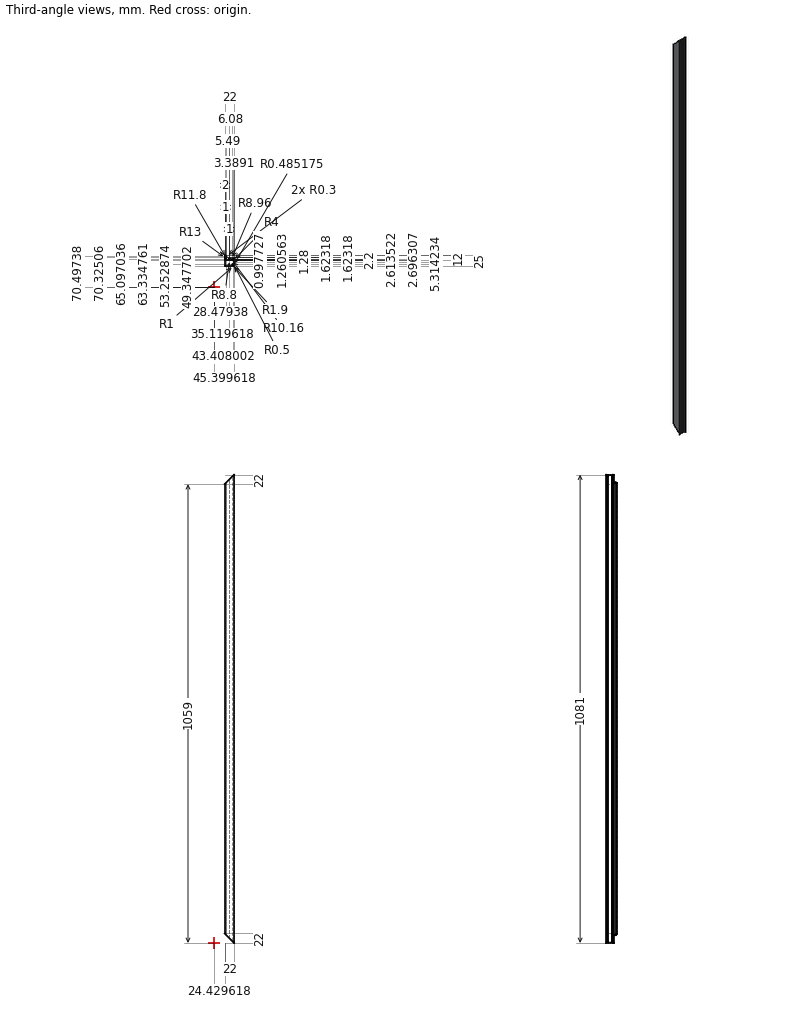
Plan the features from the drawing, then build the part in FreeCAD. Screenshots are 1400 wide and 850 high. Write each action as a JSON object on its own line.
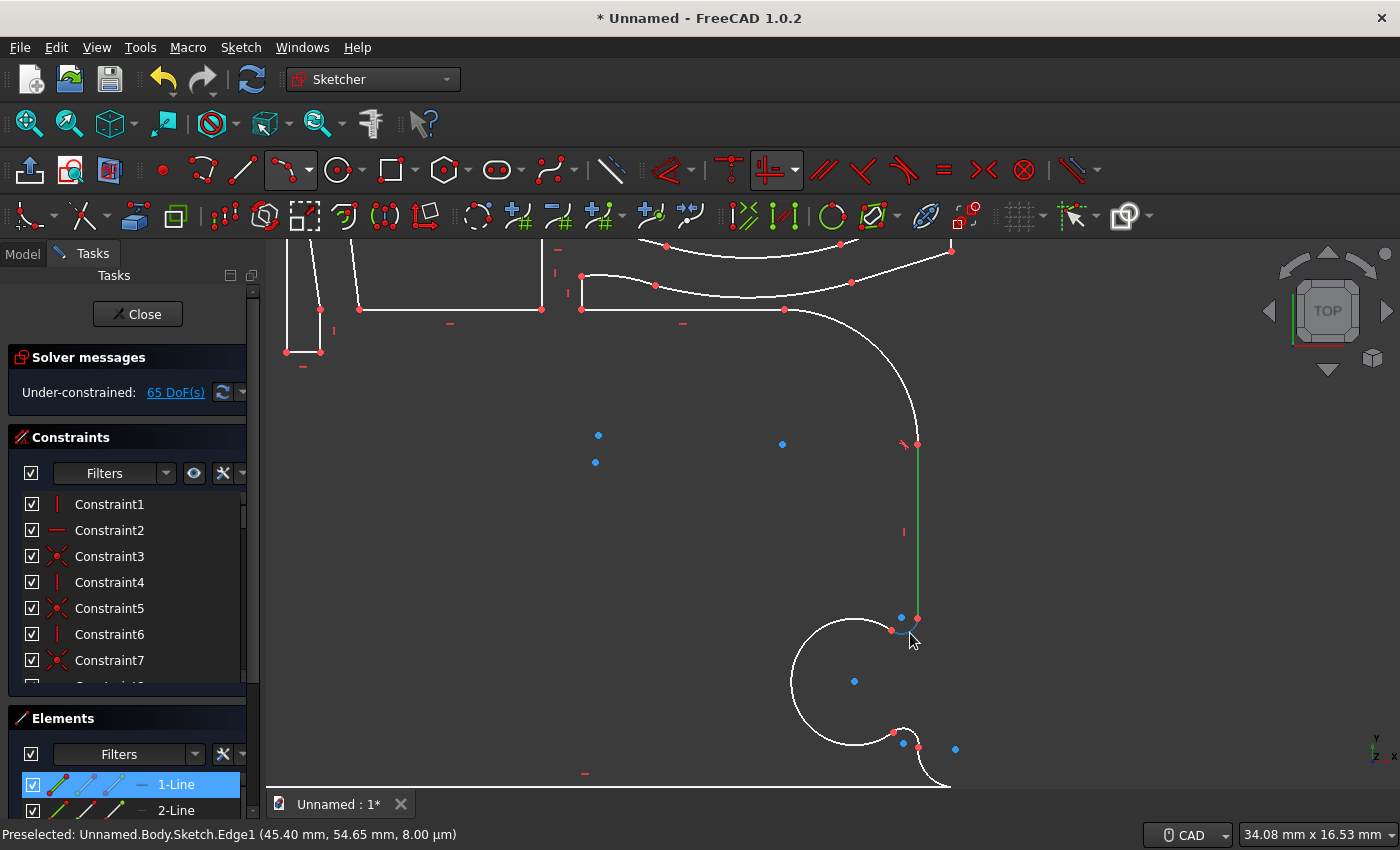
{"action": "left_click", "coordinate": [908, 632]}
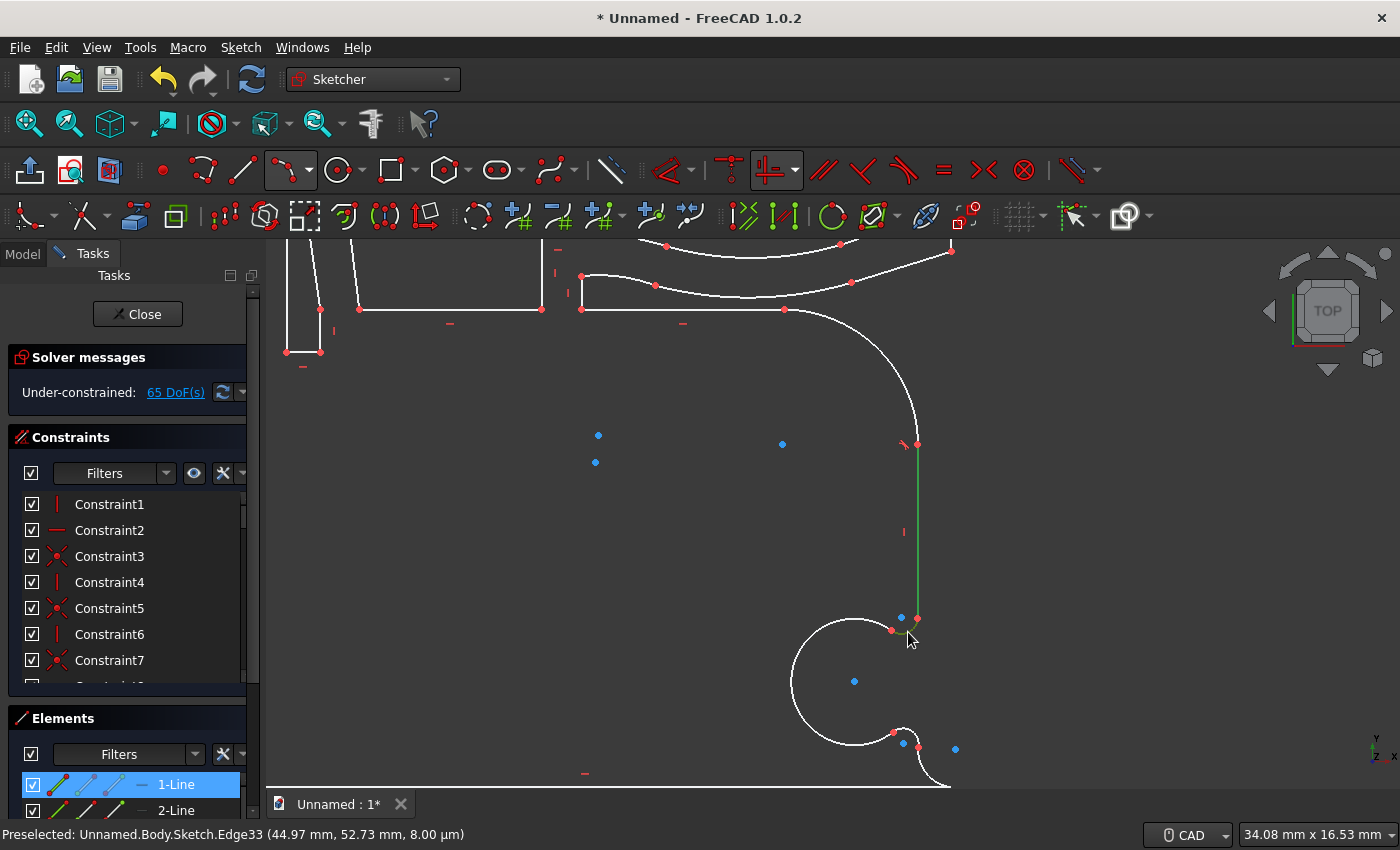
{"action": "key", "text": "t"}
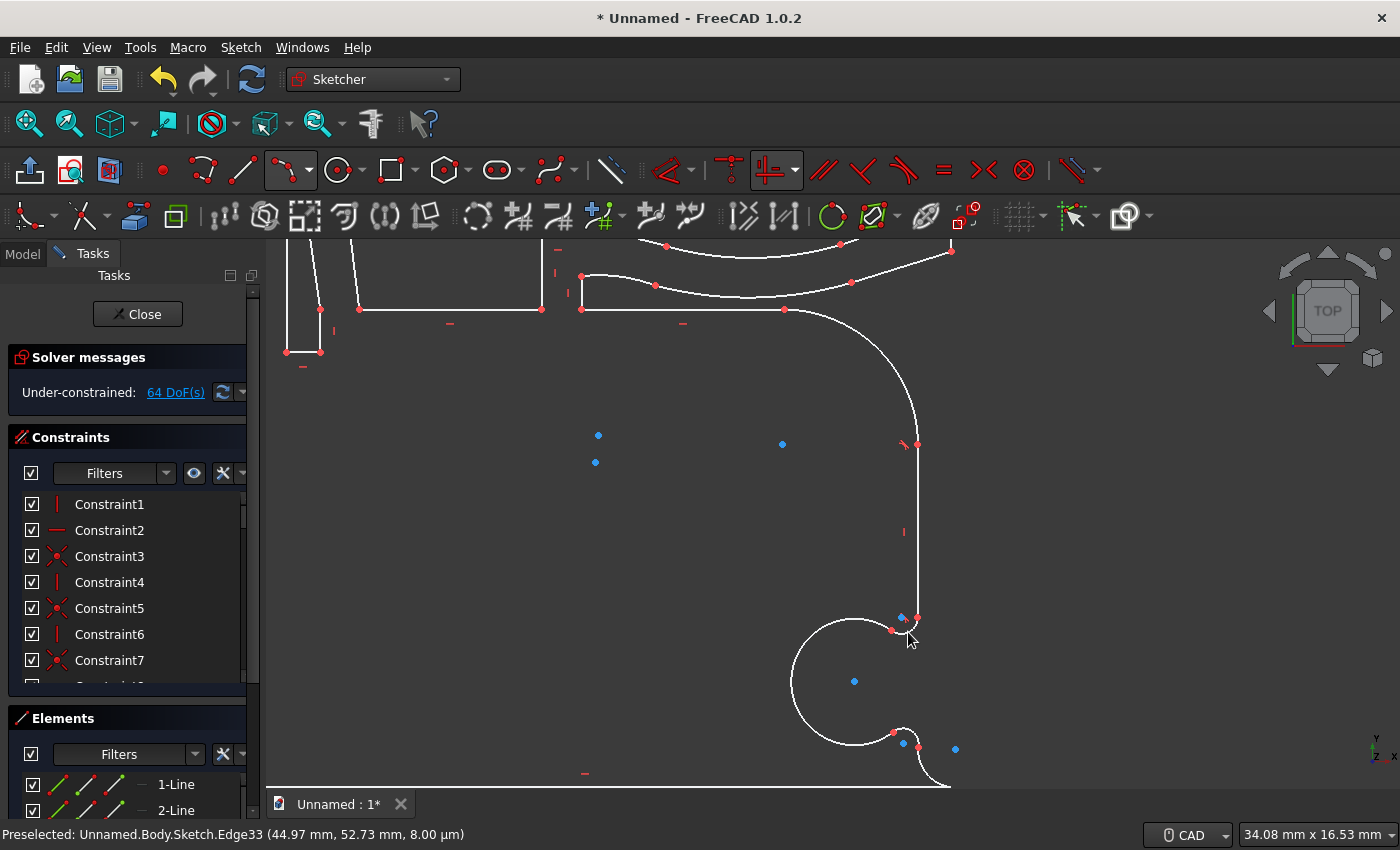
{"action": "left_click", "coordinate": [724, 310]}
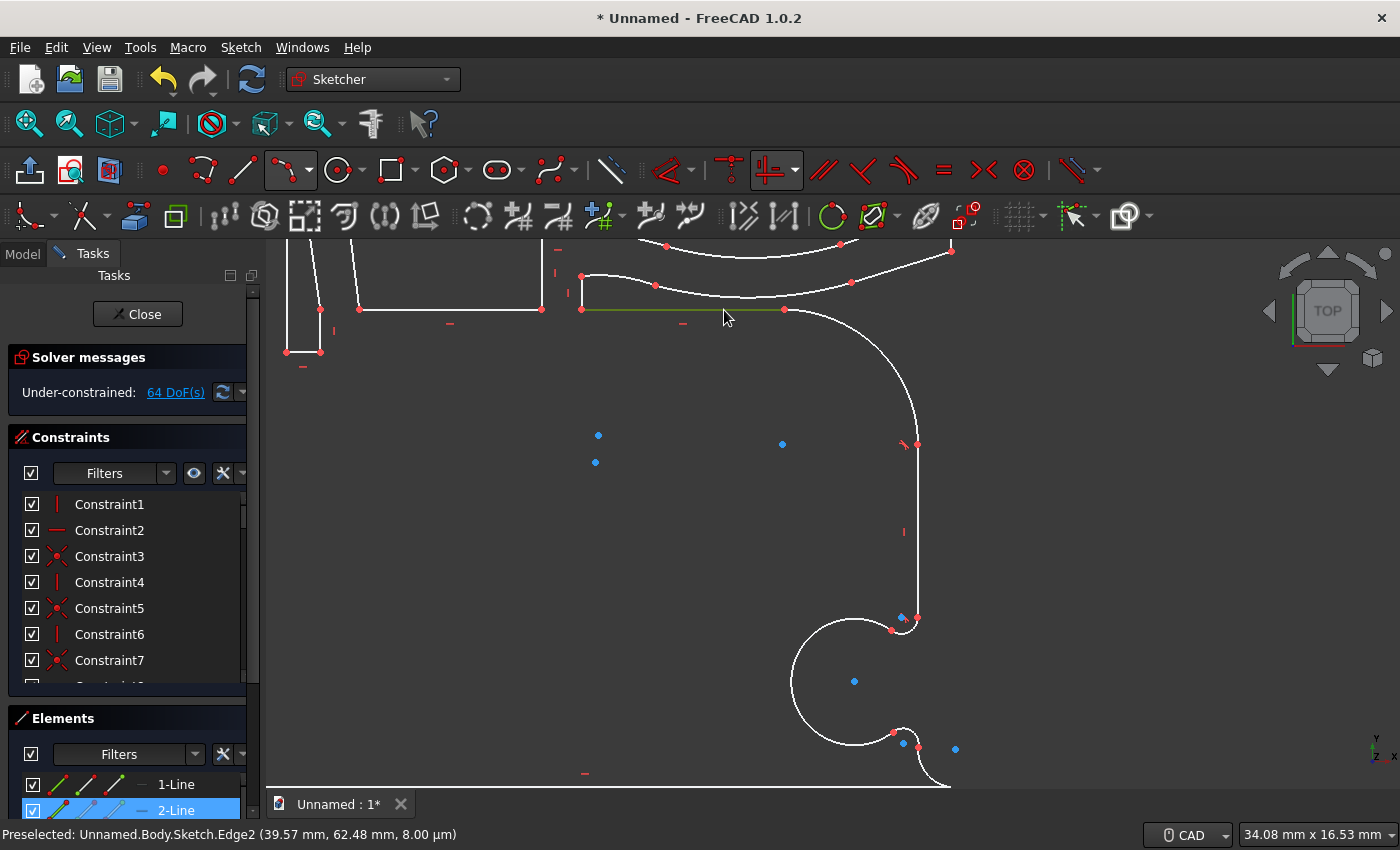
{"action": "left_click", "coordinate": [903, 384]}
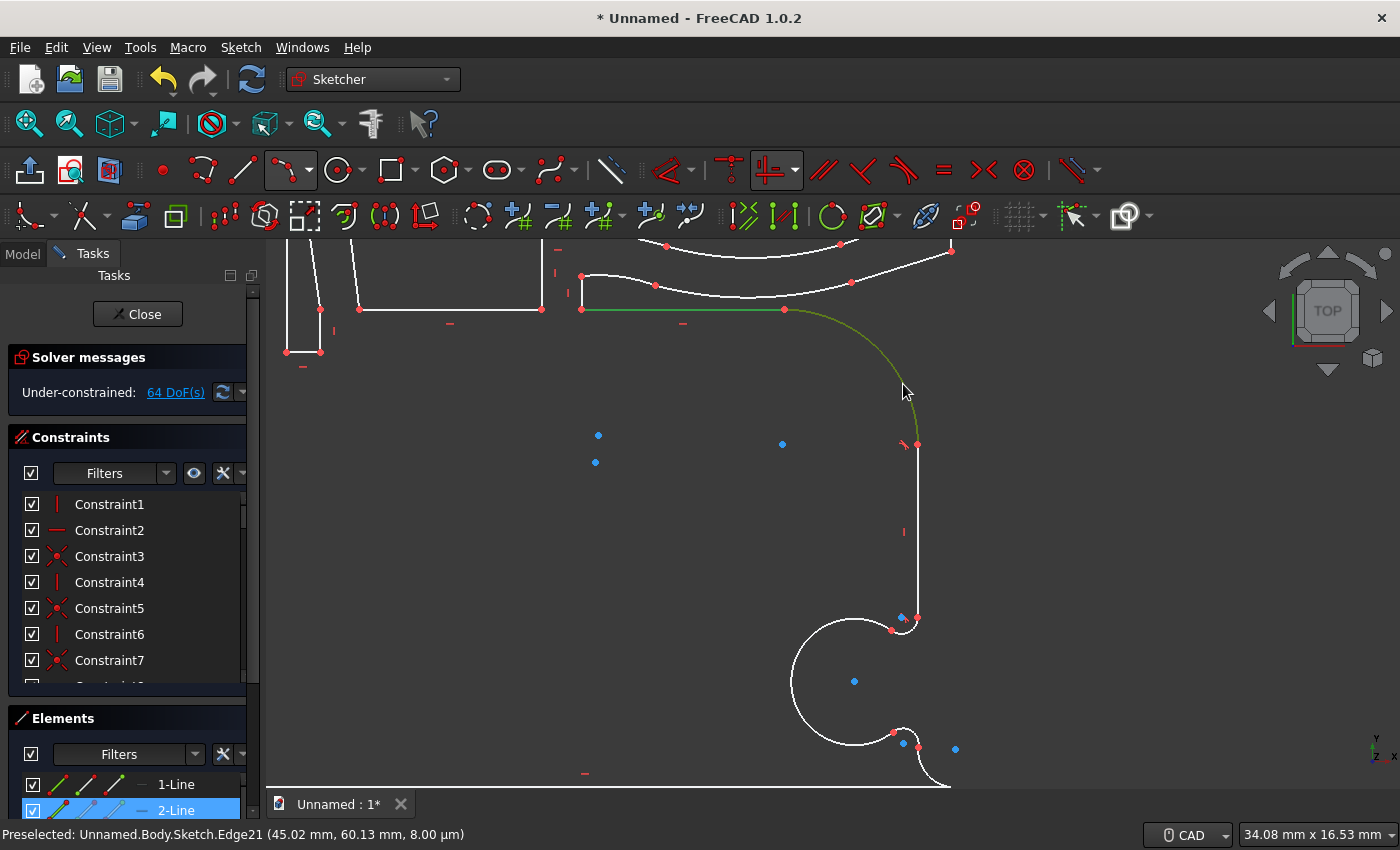
{"action": "left_click", "coordinate": [904, 170]}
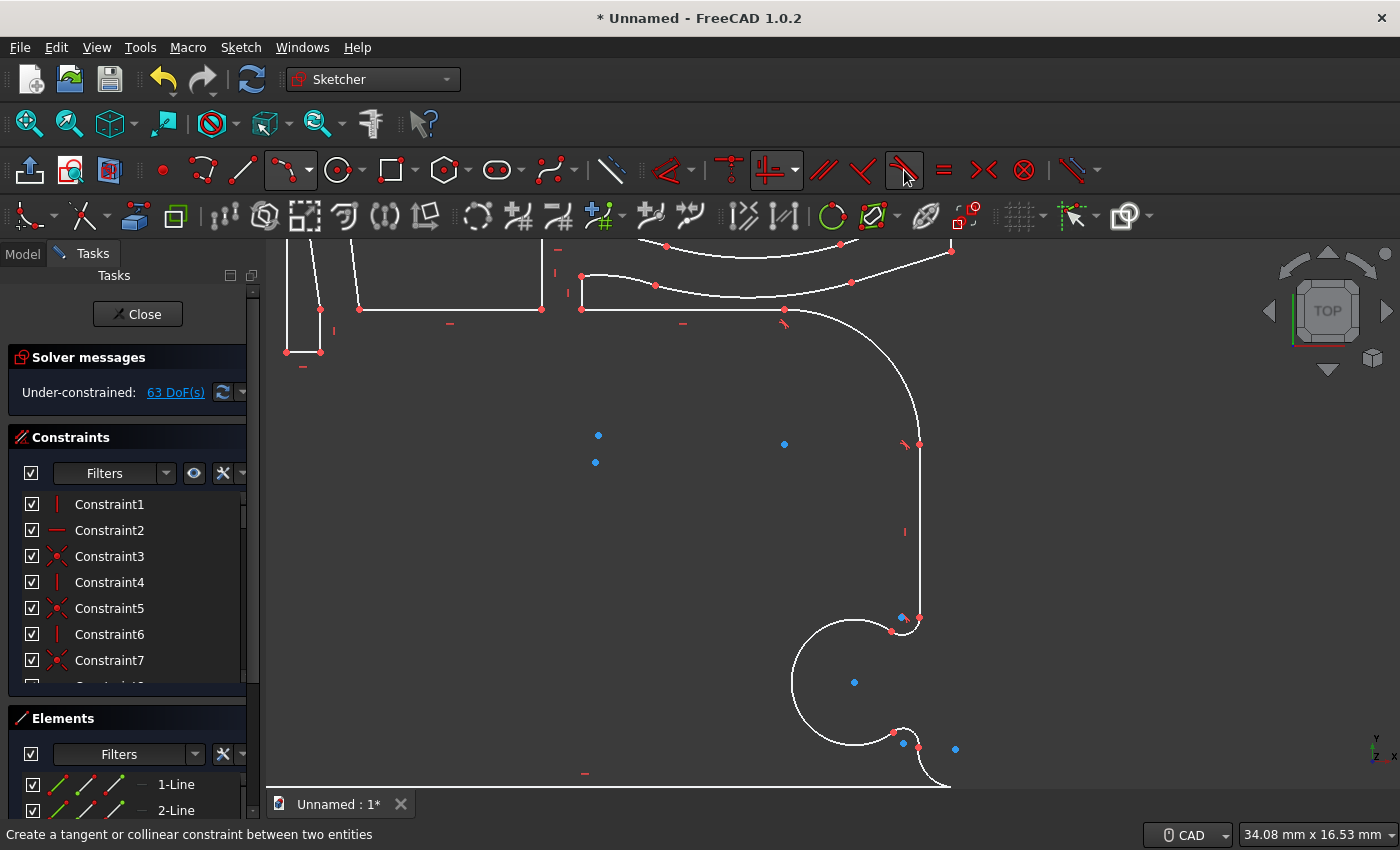
{"action": "left_click", "coordinate": [881, 273]}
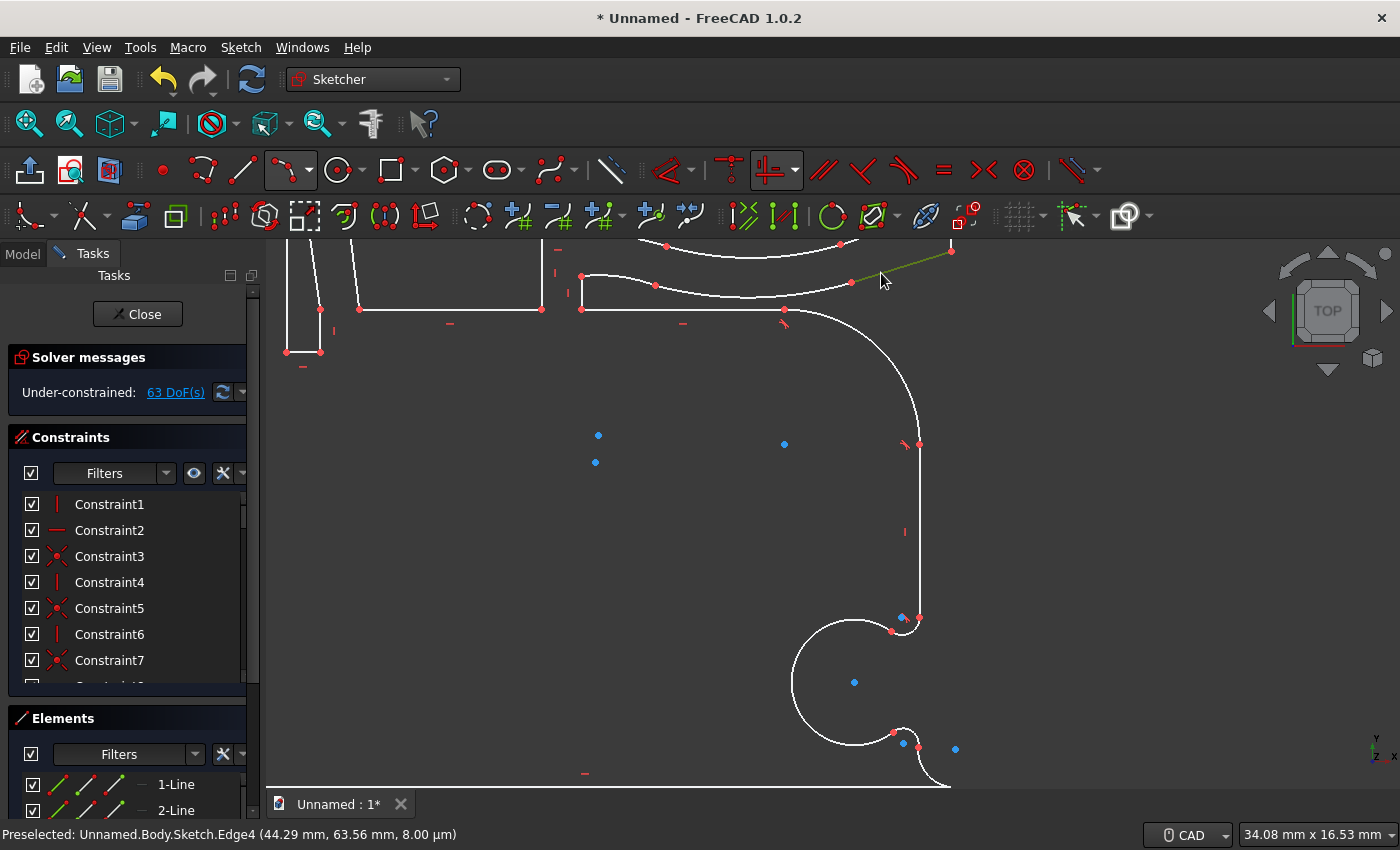
{"action": "left_click", "coordinate": [714, 296]}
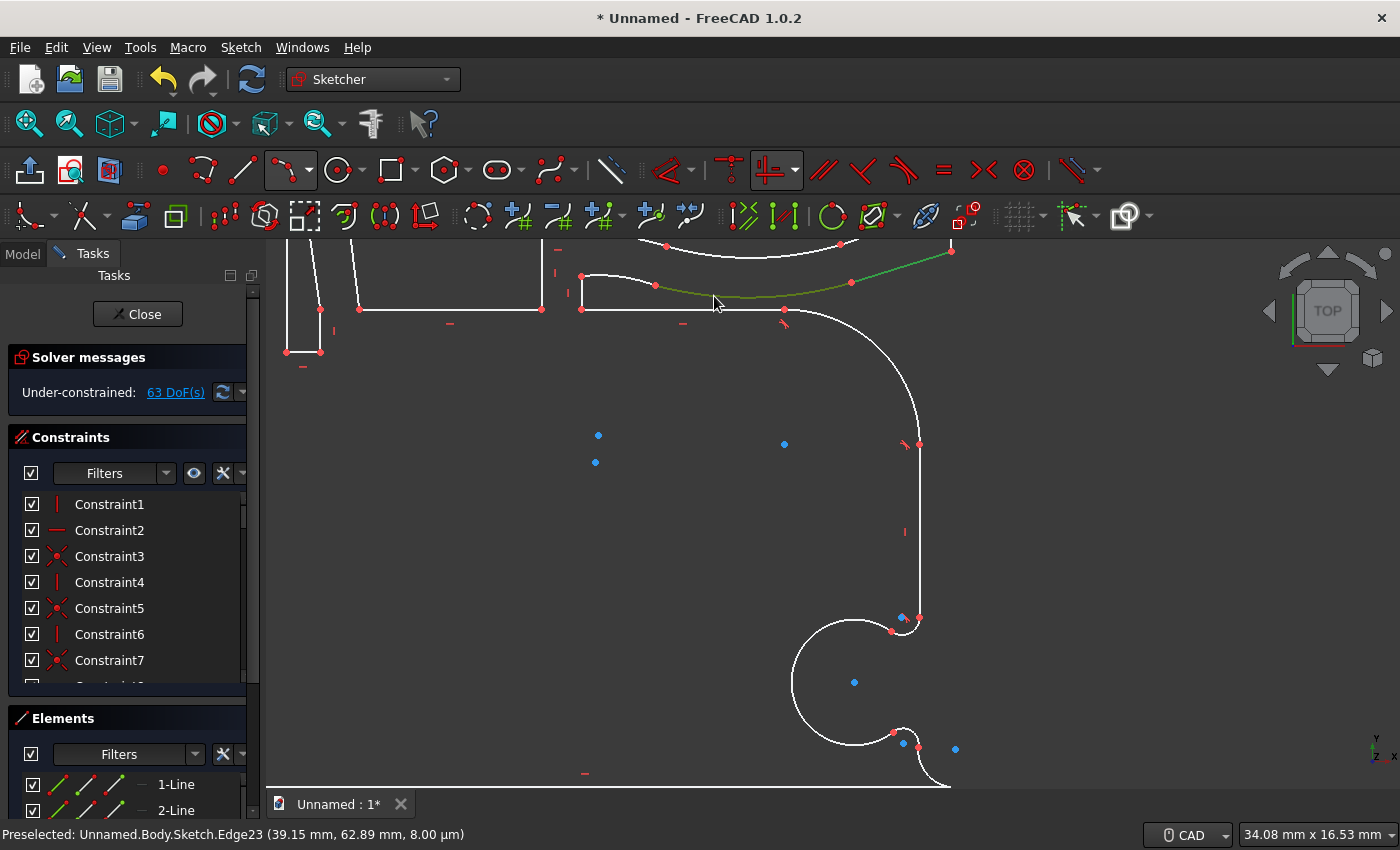
{"action": "left_click", "coordinate": [904, 170]}